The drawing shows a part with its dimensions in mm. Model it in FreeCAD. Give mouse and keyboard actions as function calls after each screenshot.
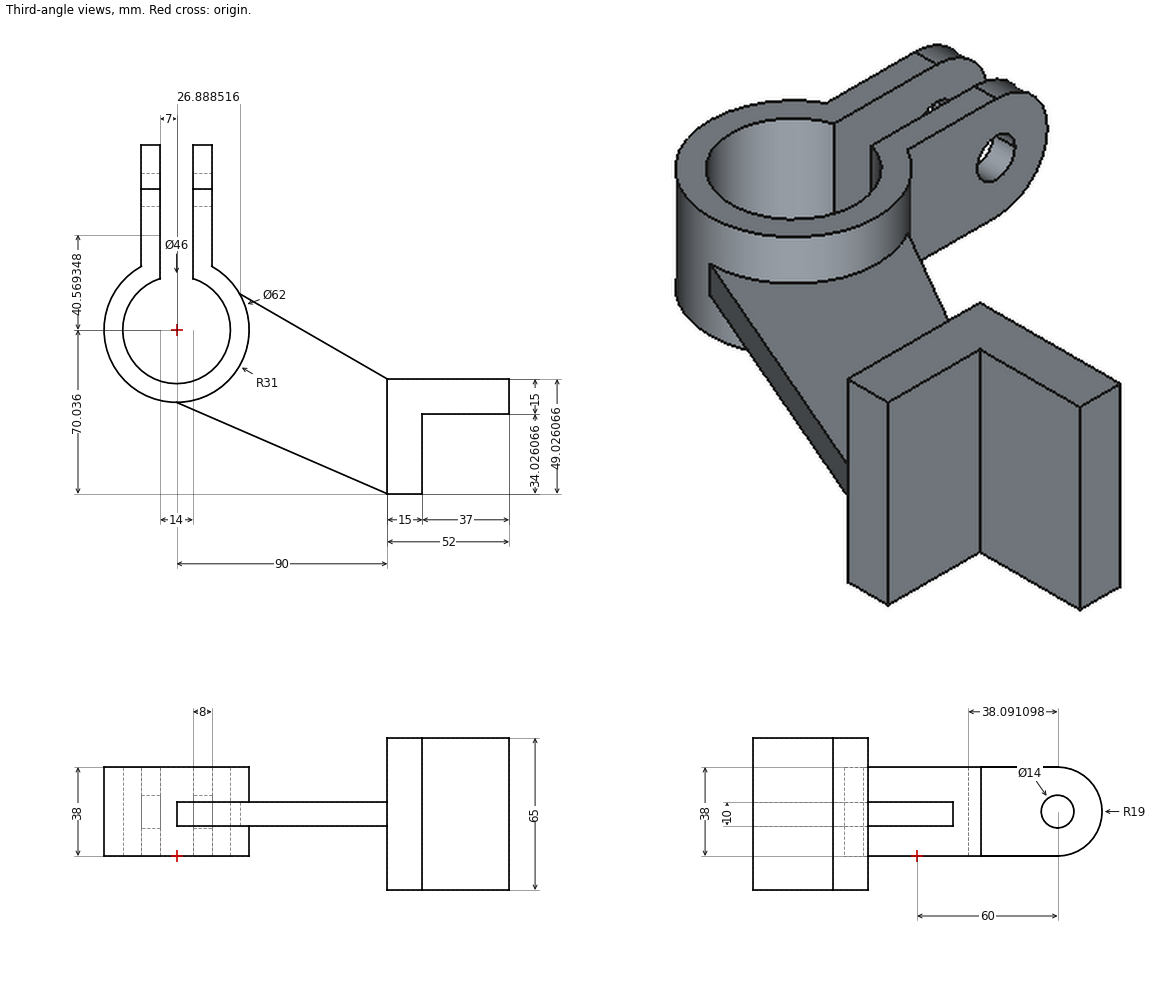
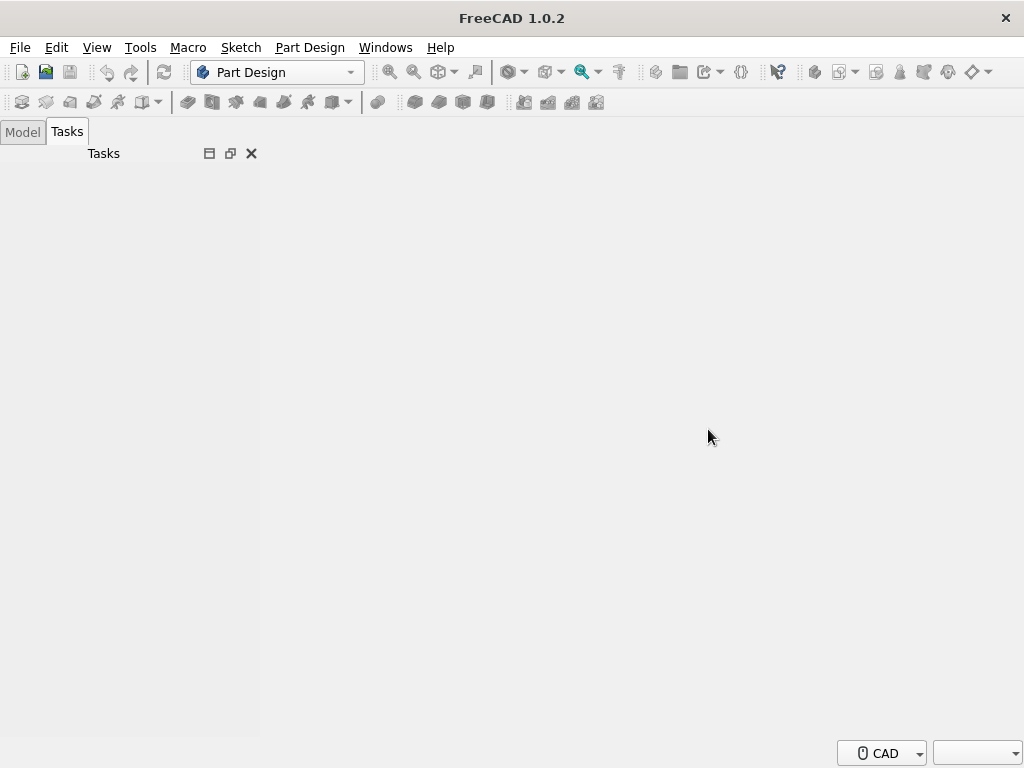
click(22, 72)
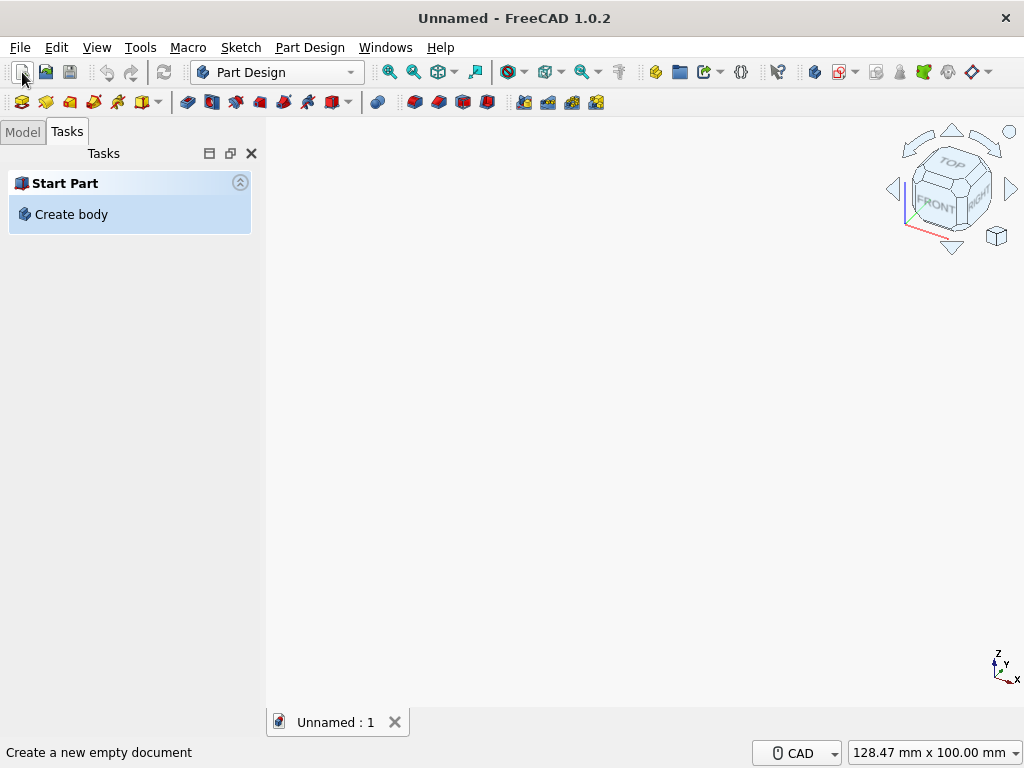
click(840, 72)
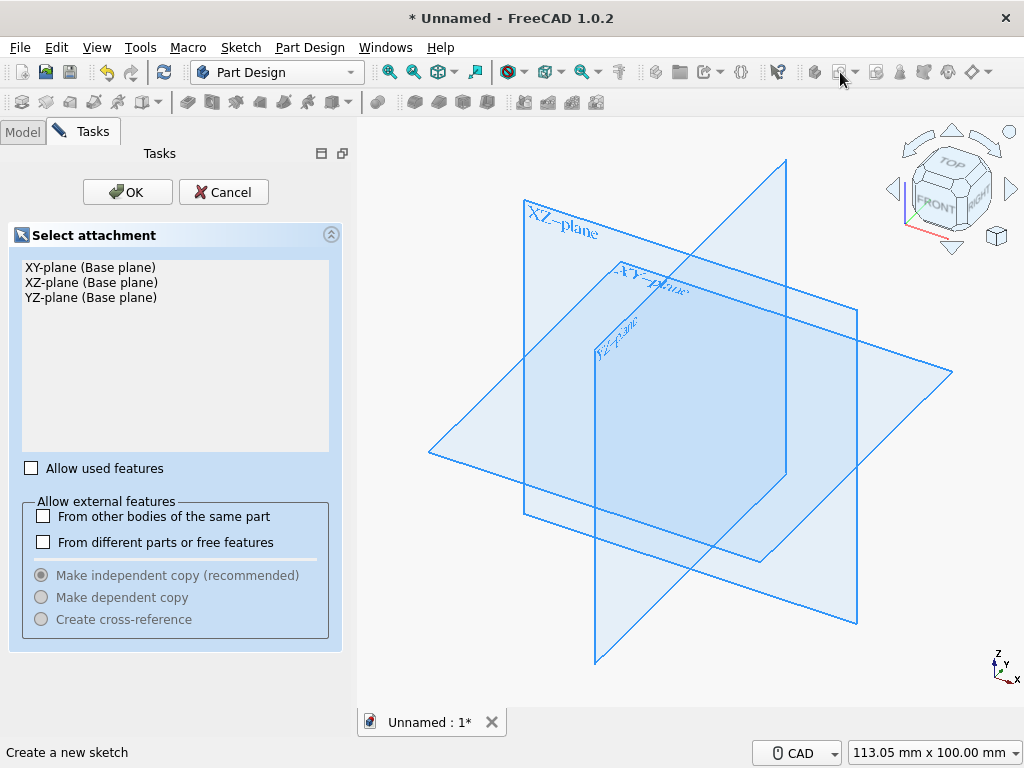
click(82, 268)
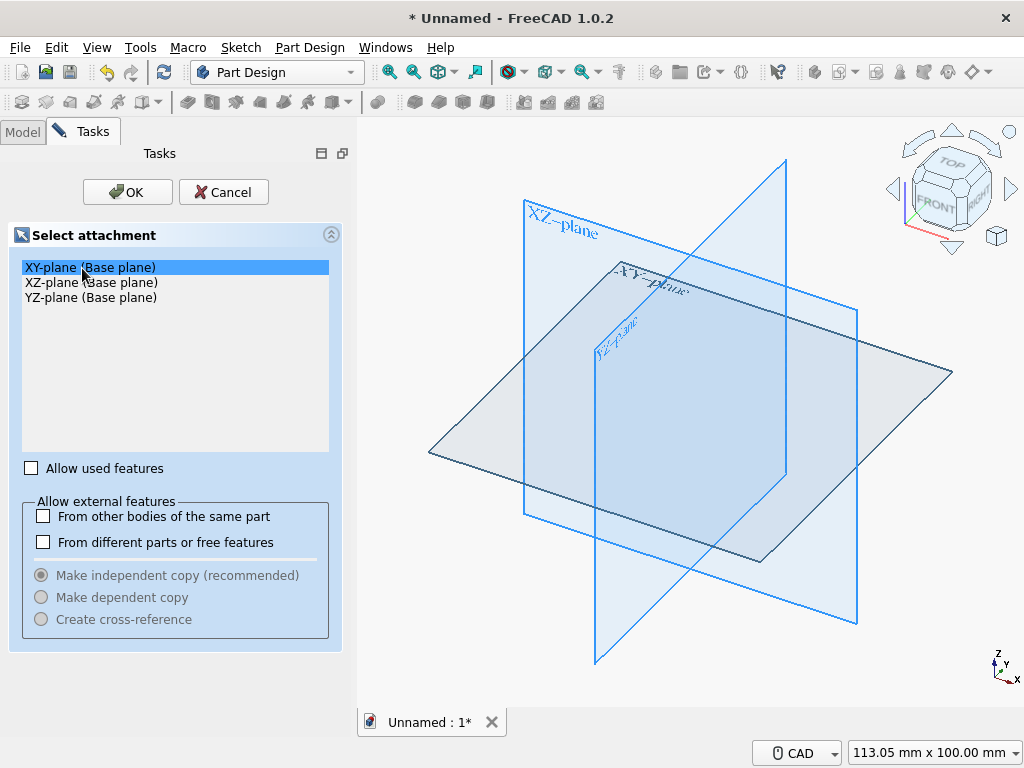
click(128, 192)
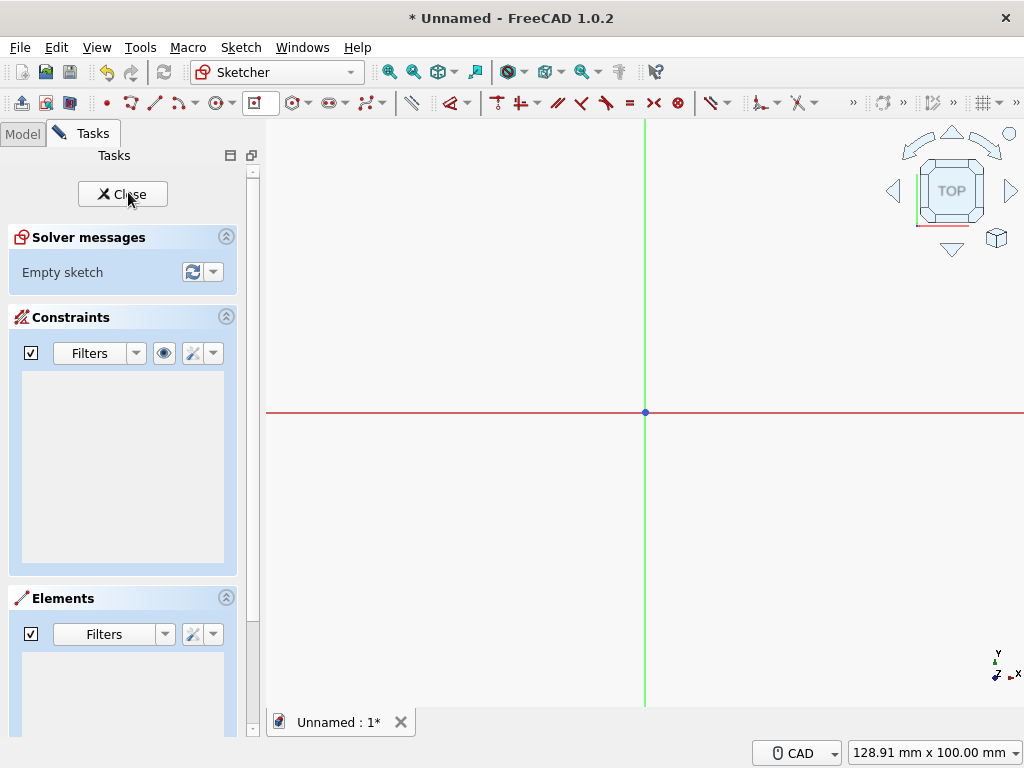
click(216, 104)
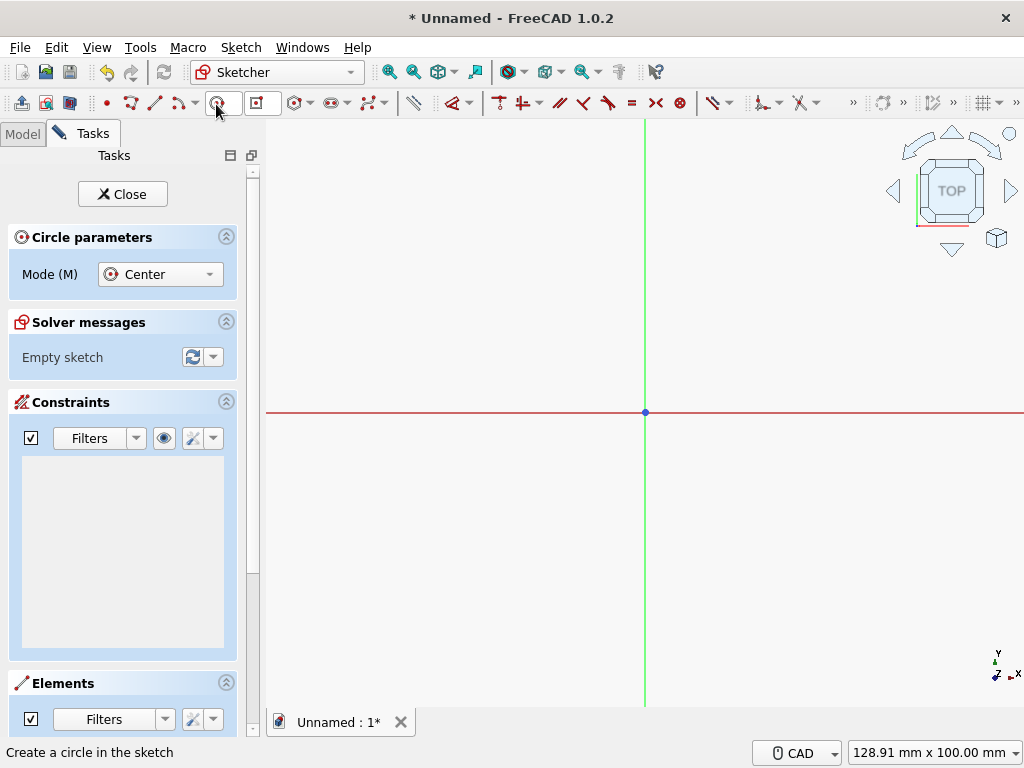
click(645, 413)
move(774, 284)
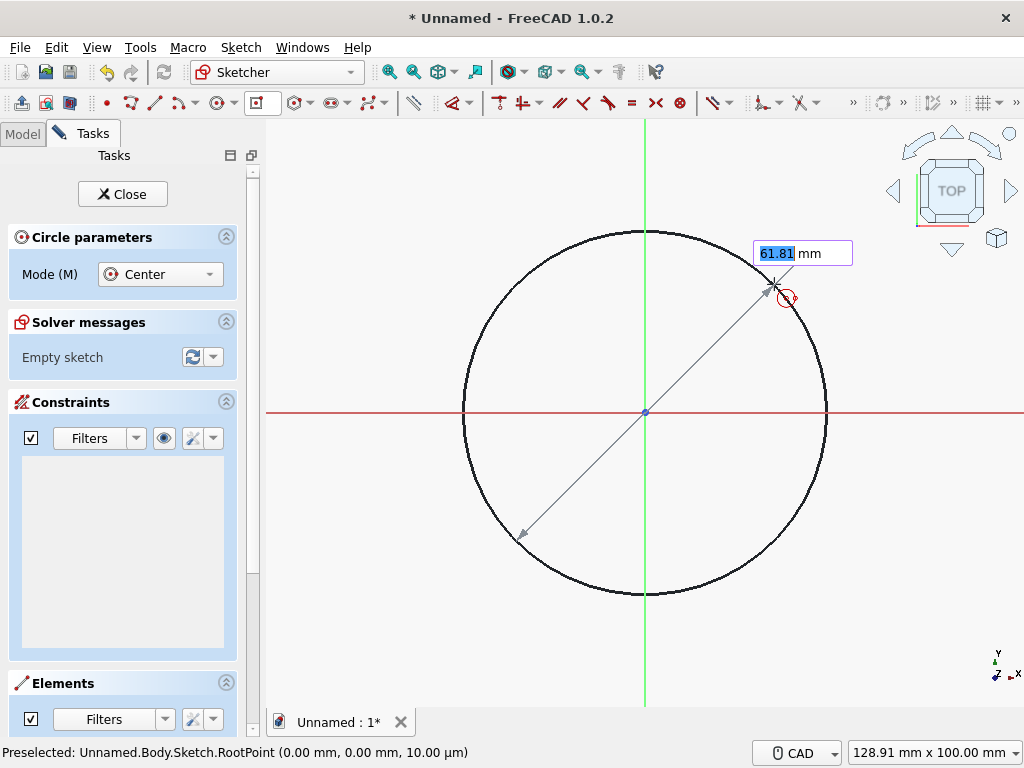
text(62)
key(Return)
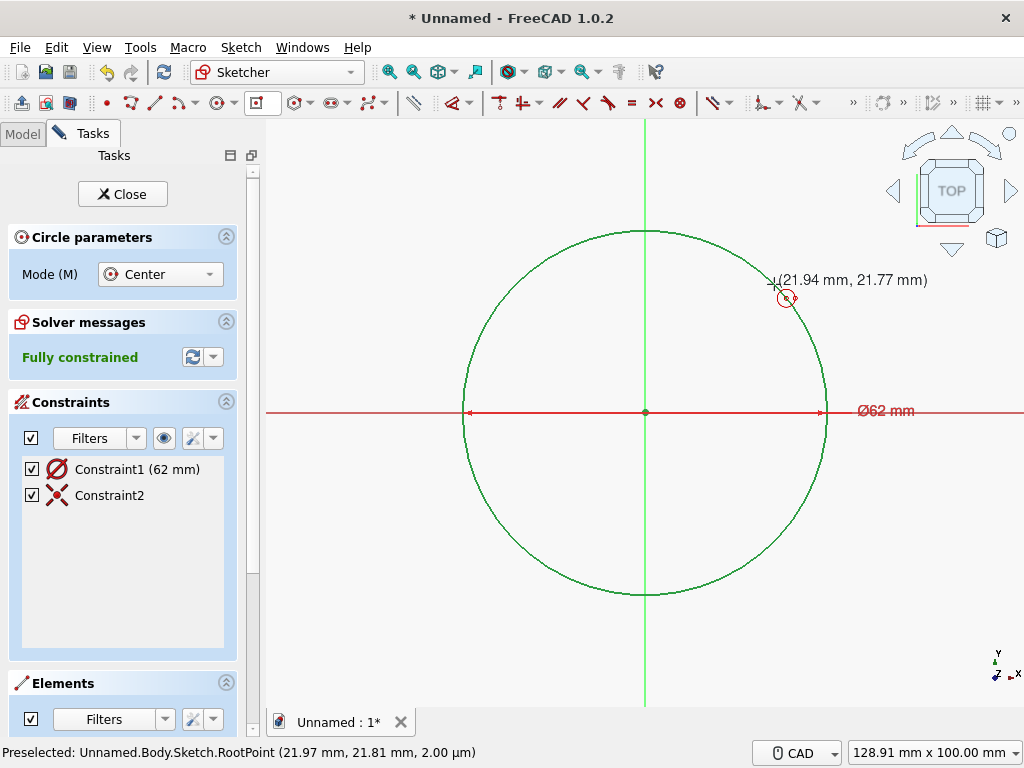
click(645, 413)
move(741, 317)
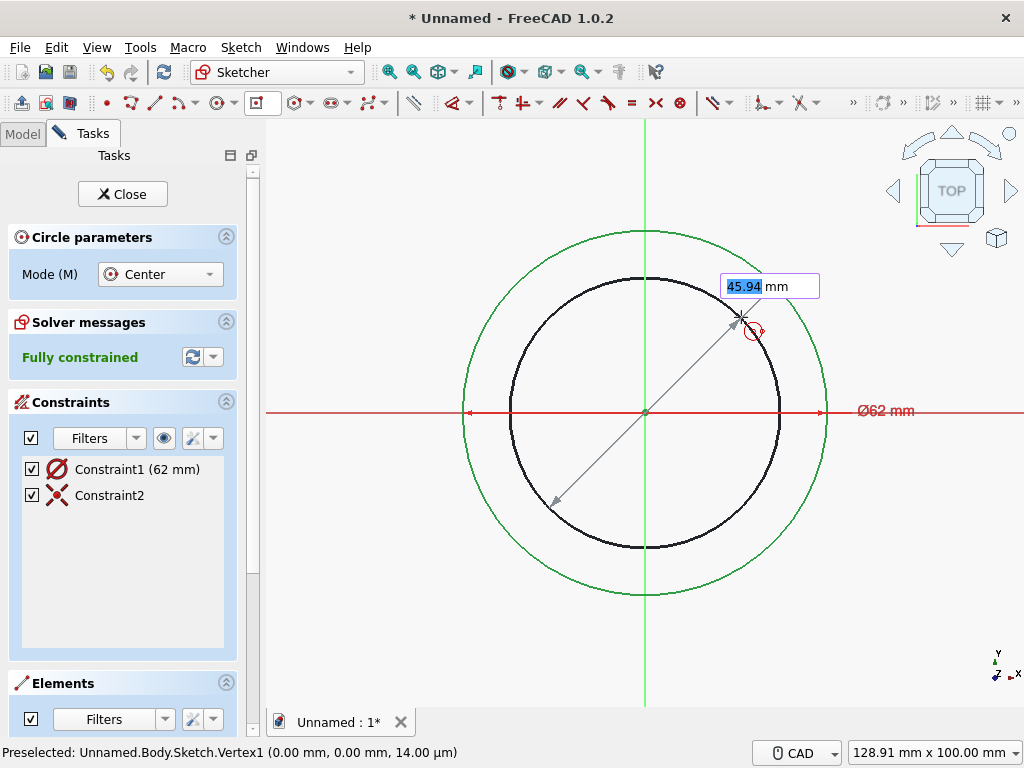
text(46)
key(Return)
key(Escape)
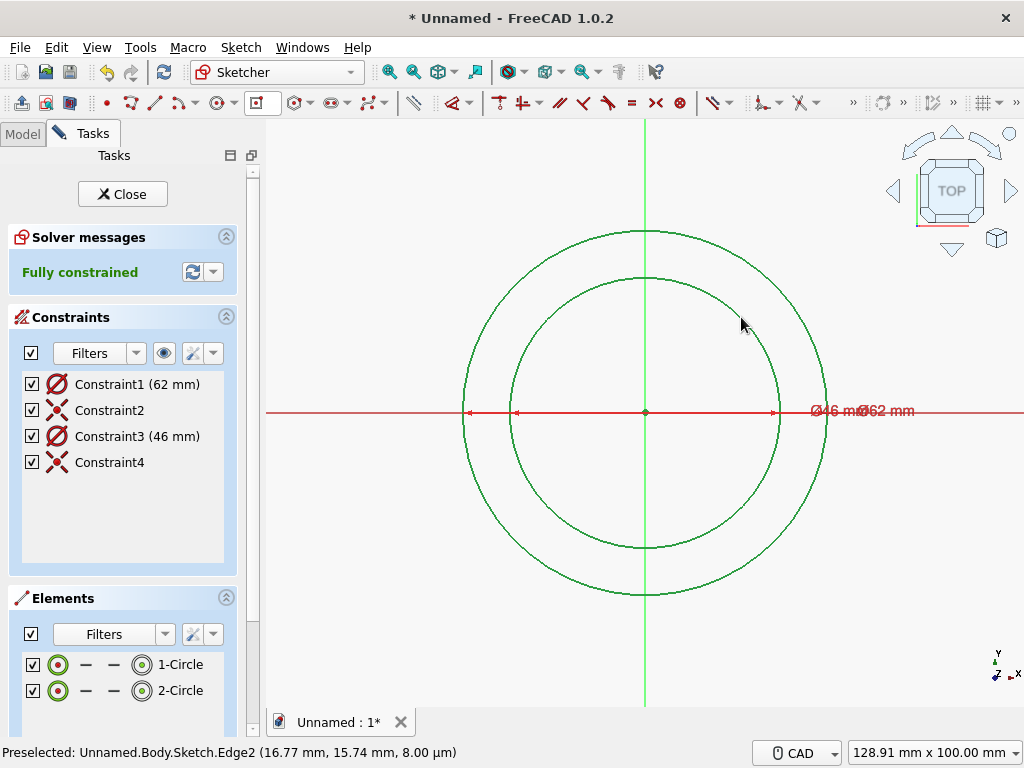
click(123, 194)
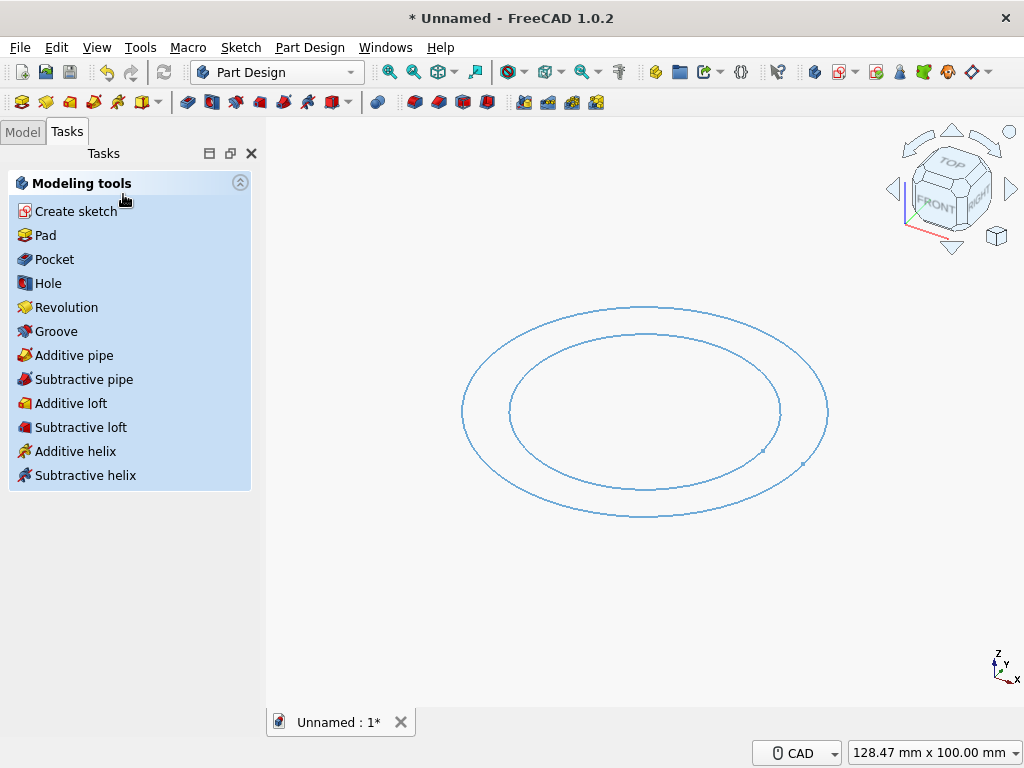
click(22, 102)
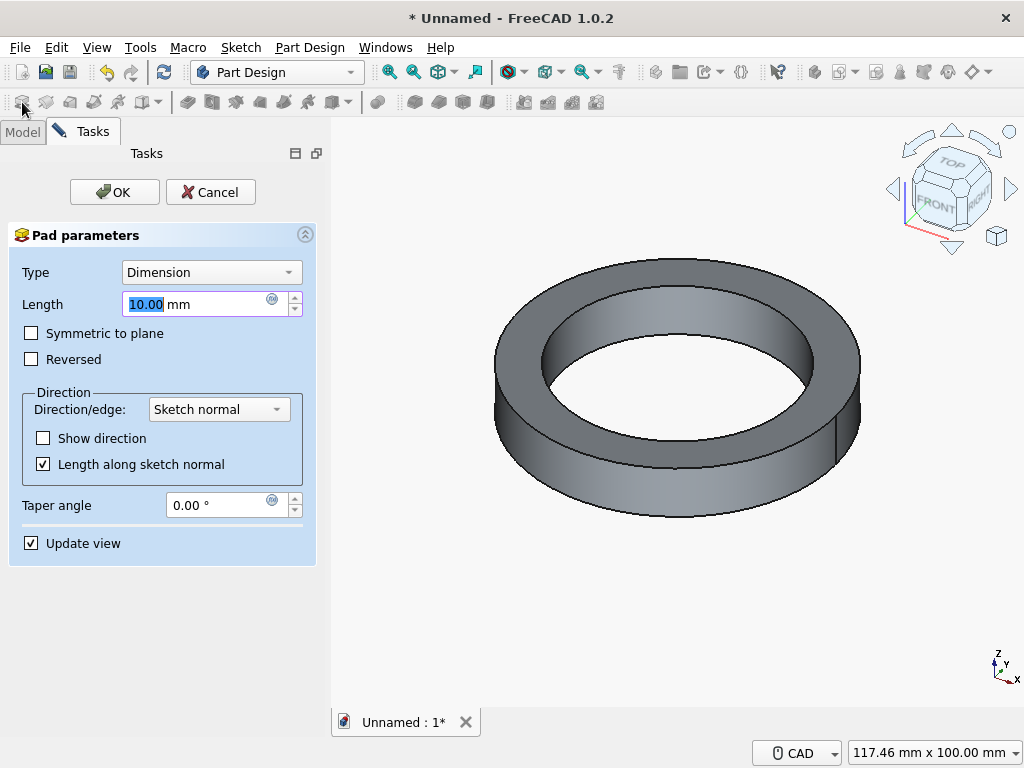
text(38)
key(Tab)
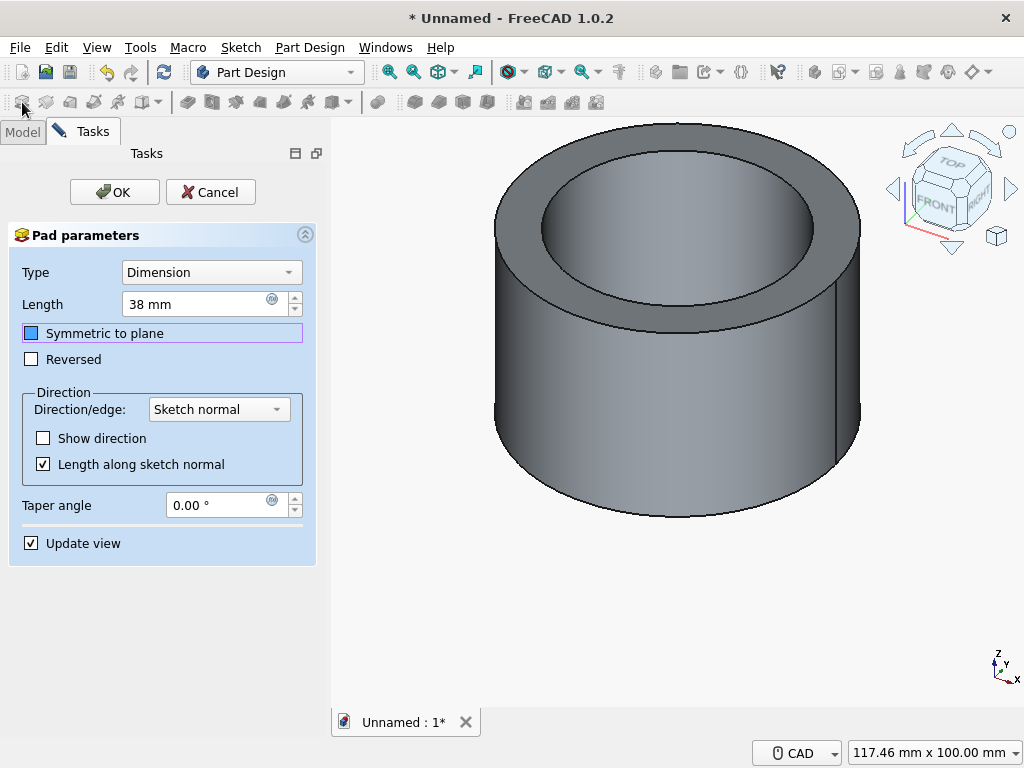
click(115, 192)